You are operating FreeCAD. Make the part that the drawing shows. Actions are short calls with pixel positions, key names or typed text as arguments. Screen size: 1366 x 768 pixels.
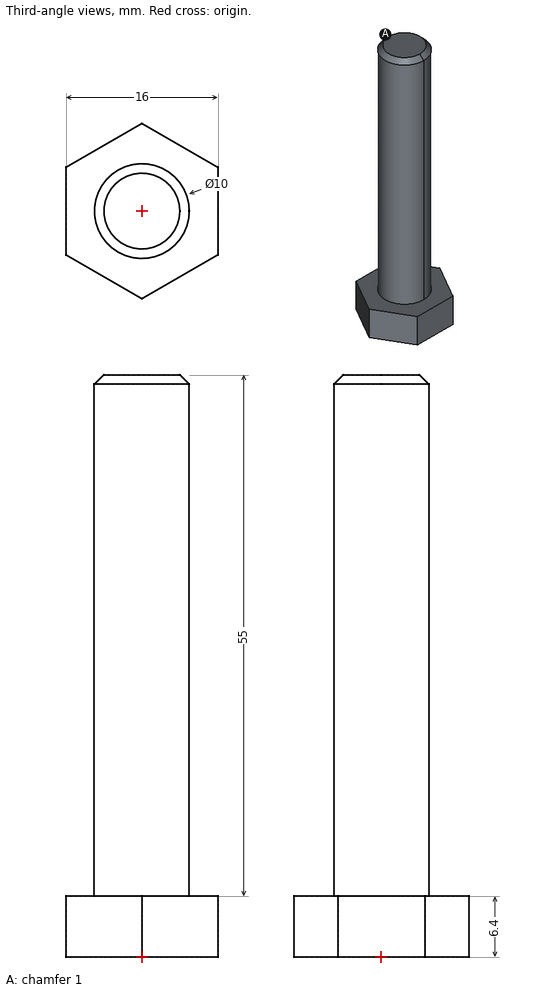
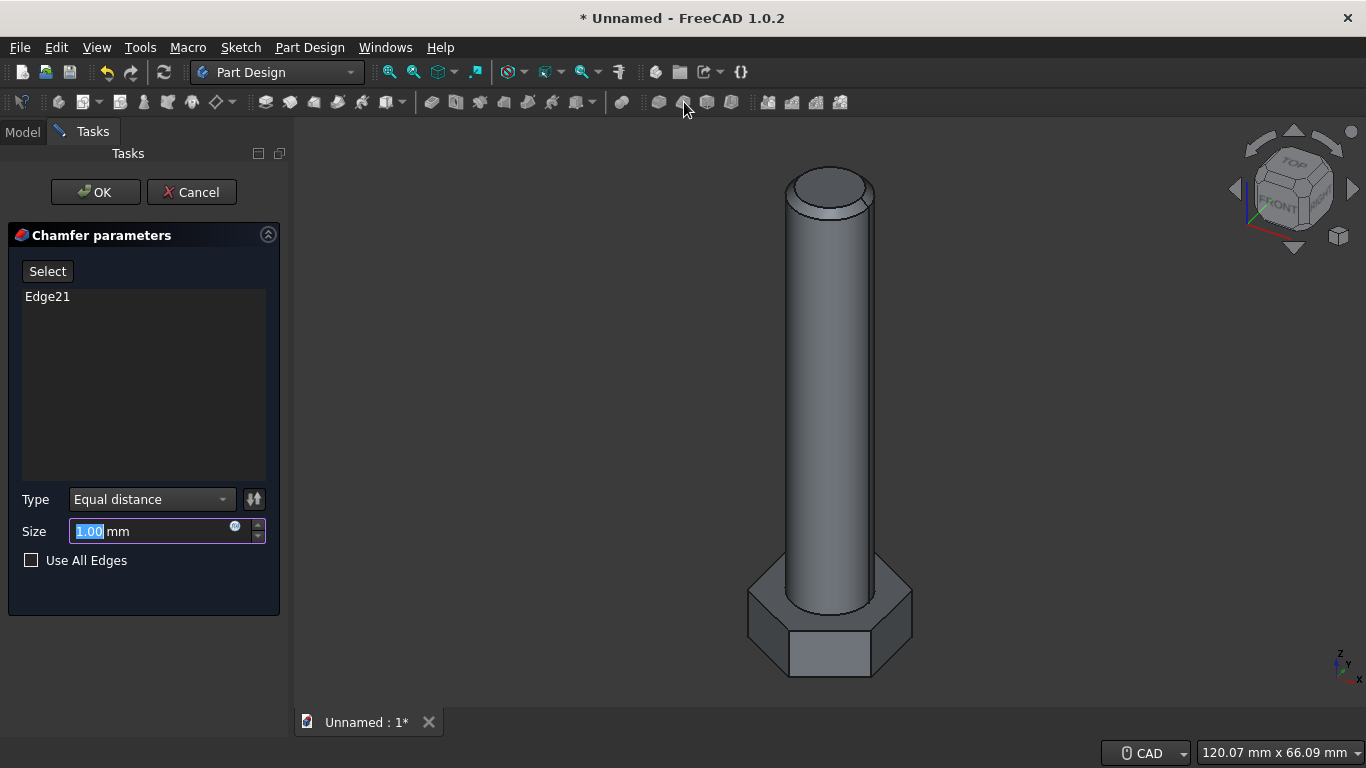
text(1)
key(Tab)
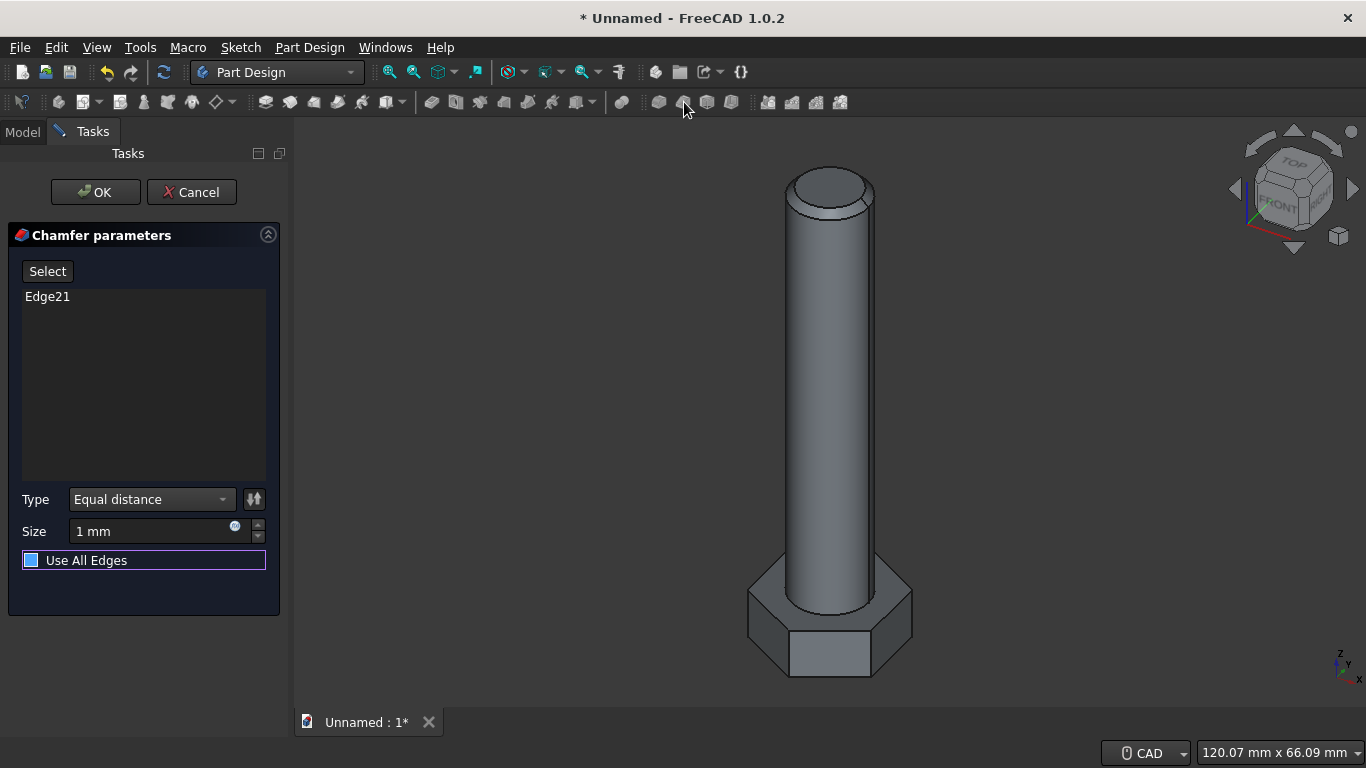
click(96, 192)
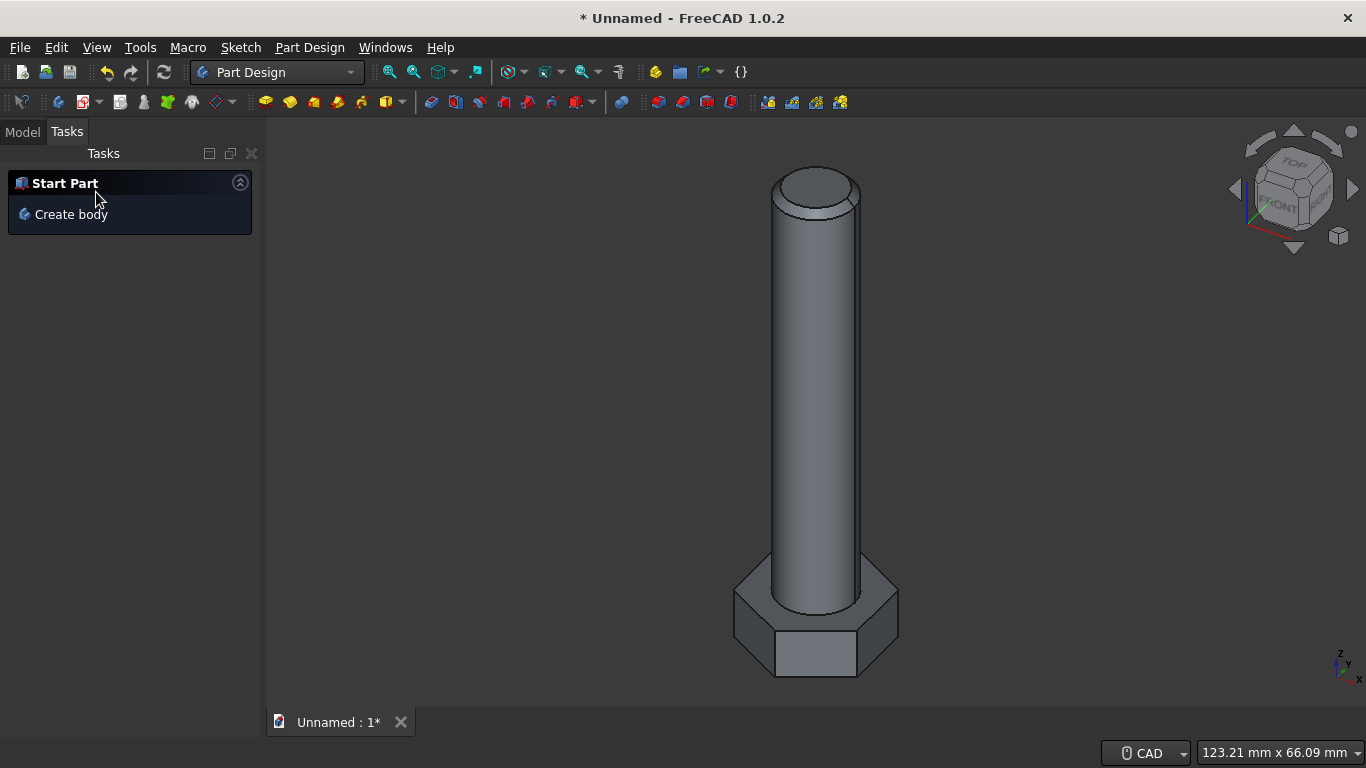
key(0)